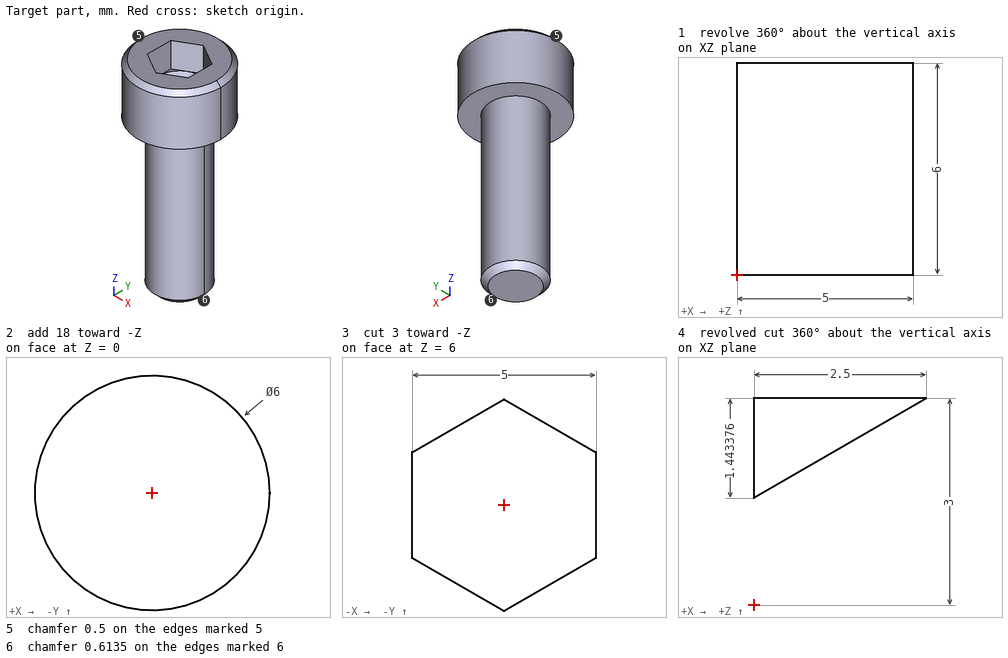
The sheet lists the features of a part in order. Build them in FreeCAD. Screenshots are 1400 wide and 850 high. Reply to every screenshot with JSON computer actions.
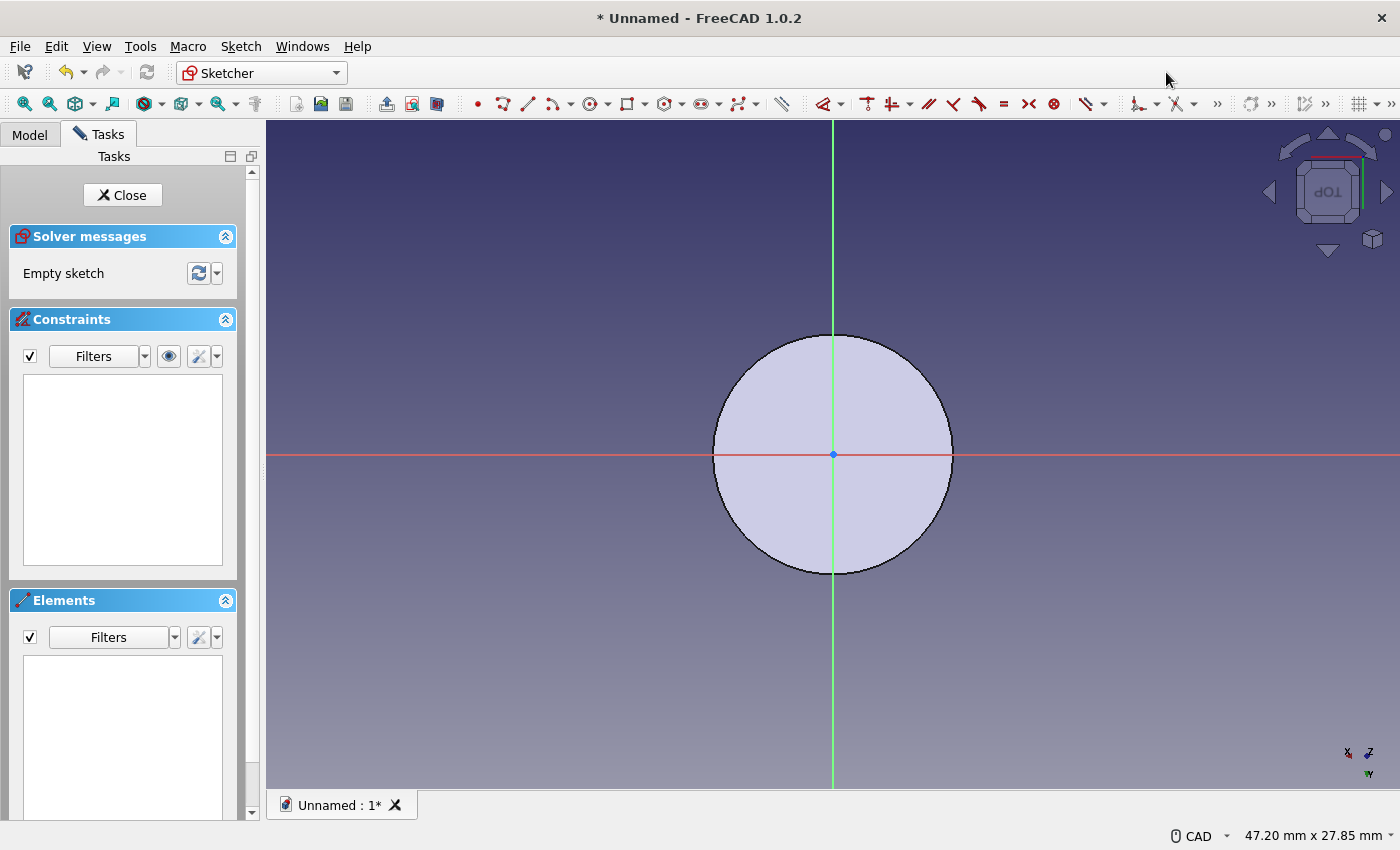
{"action": "scroll", "coordinate": [863, 454], "scroll_direction": "up", "scroll_amount": 6}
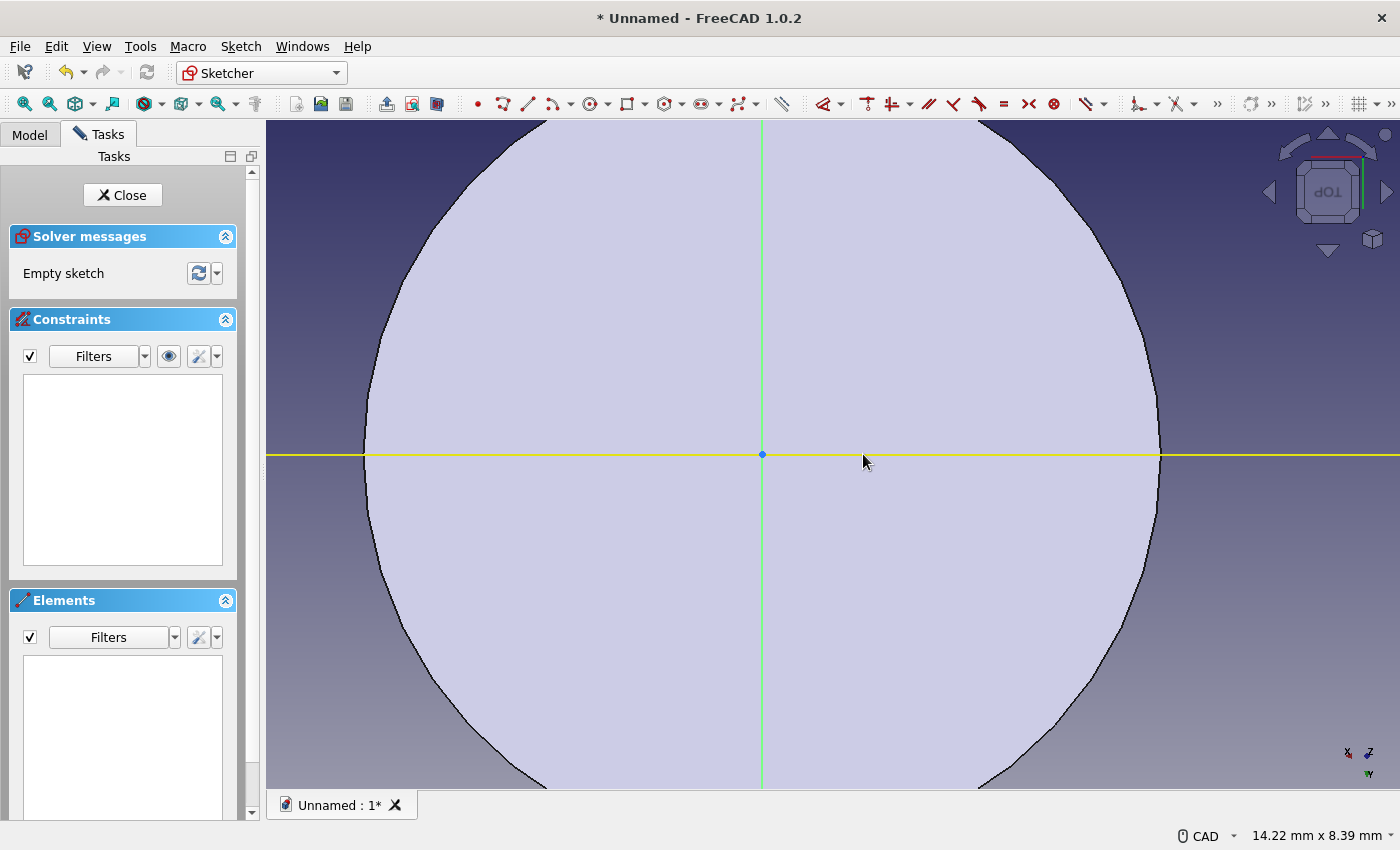
{"action": "left_click", "coordinate": [664, 104]}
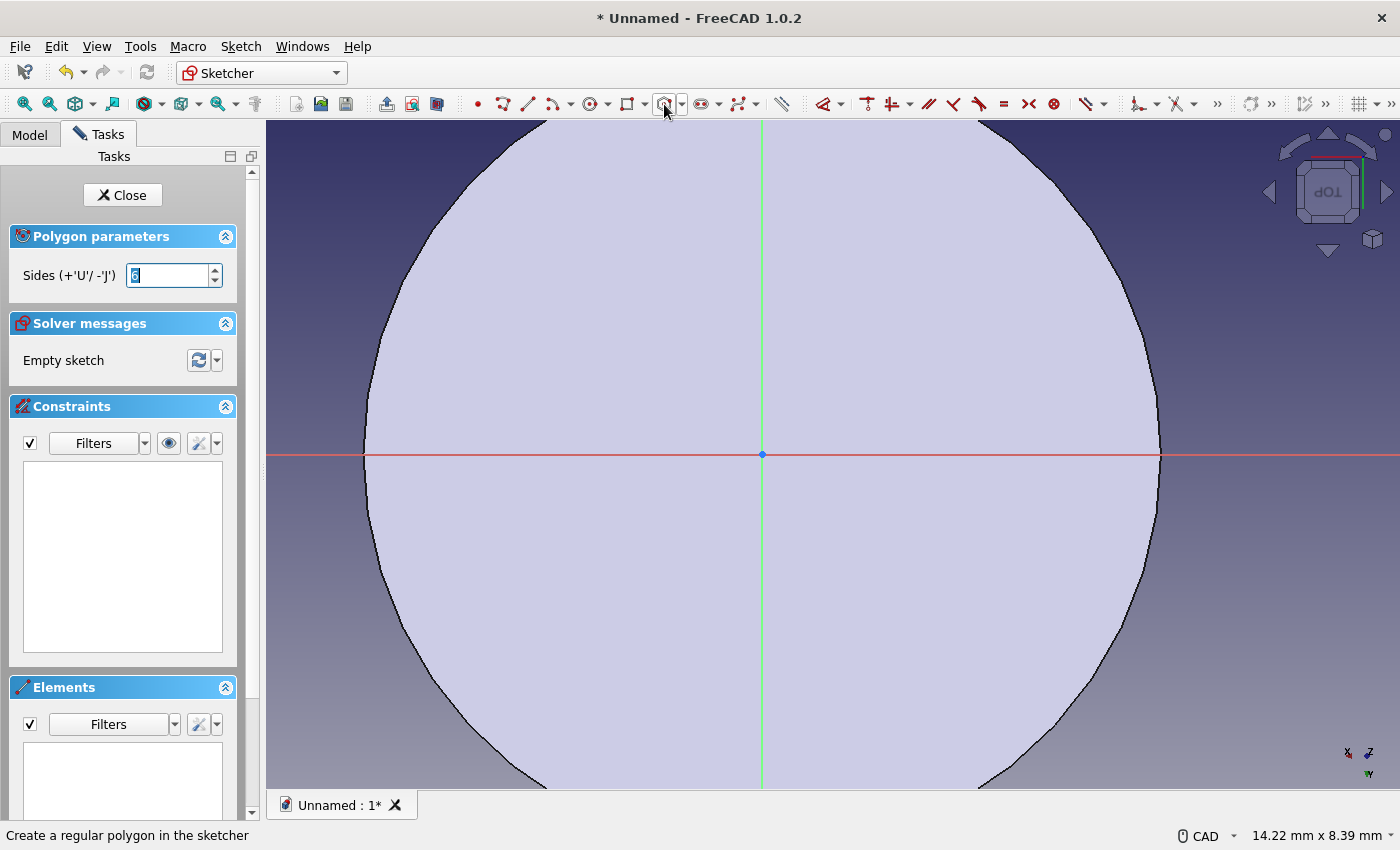
{"action": "left_click", "coordinate": [762, 454]}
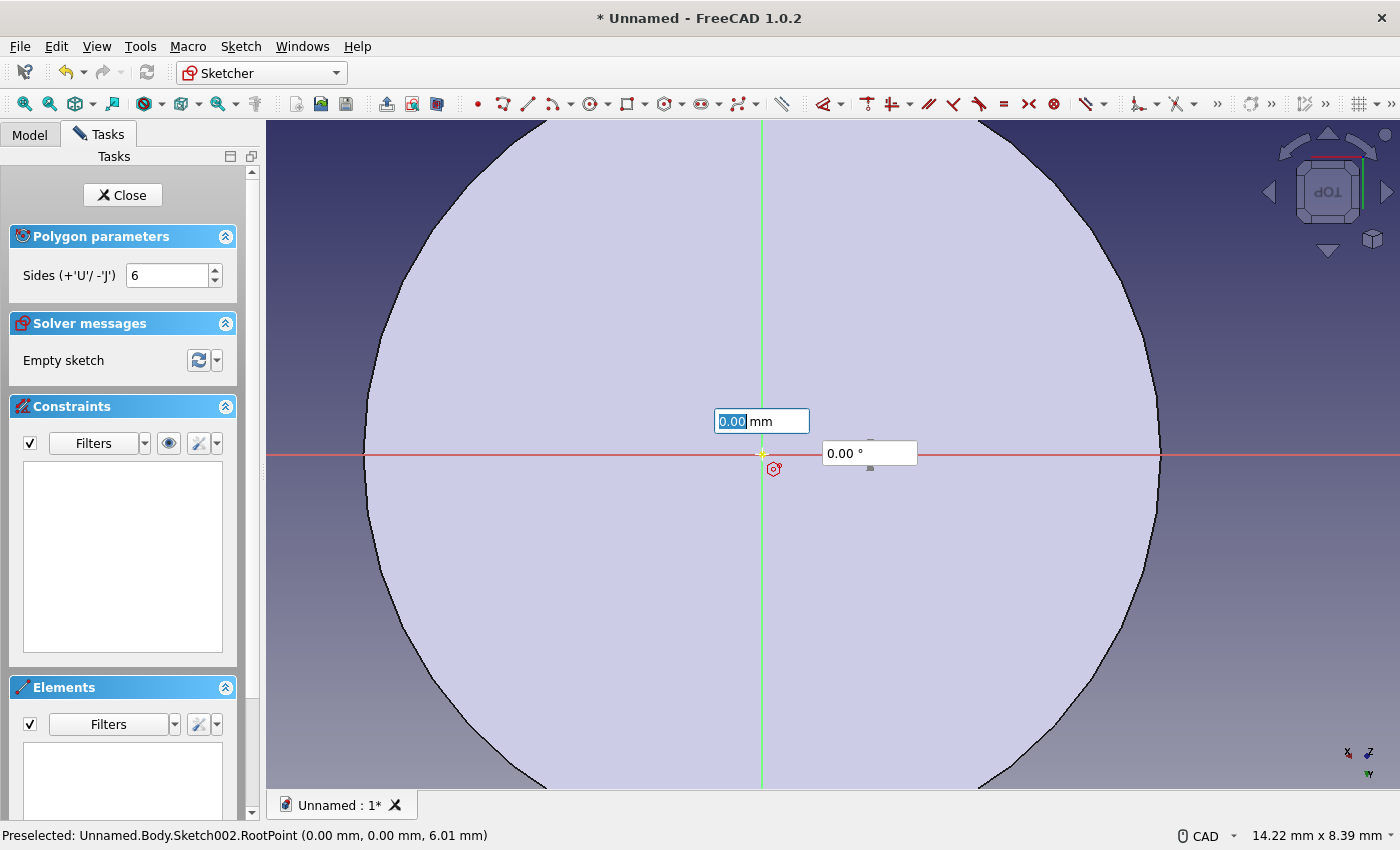
{"action": "left_click", "coordinate": [762, 685]}
{"action": "right_click", "coordinate": [762, 685]}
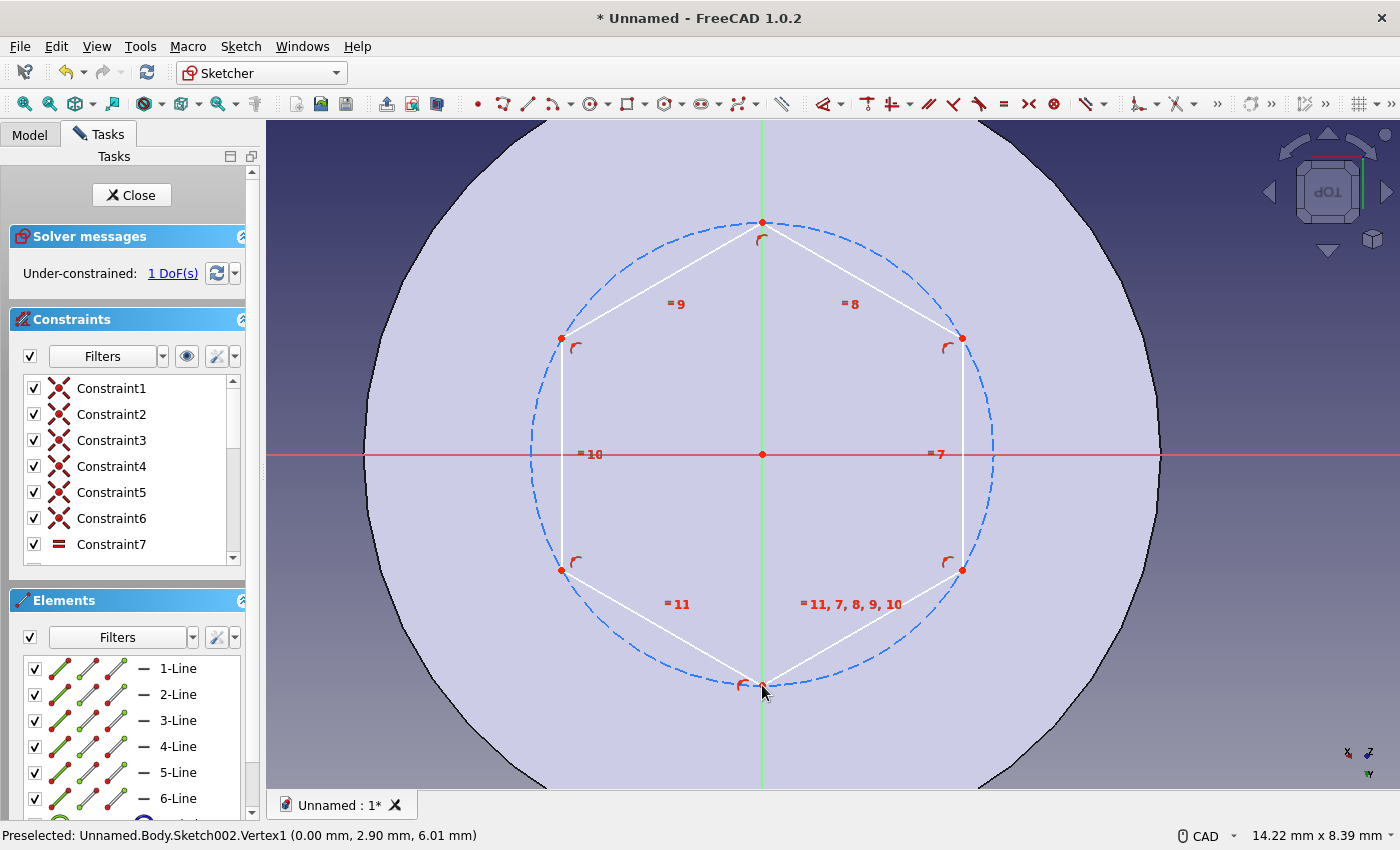
{"action": "left_click", "coordinate": [822, 104]}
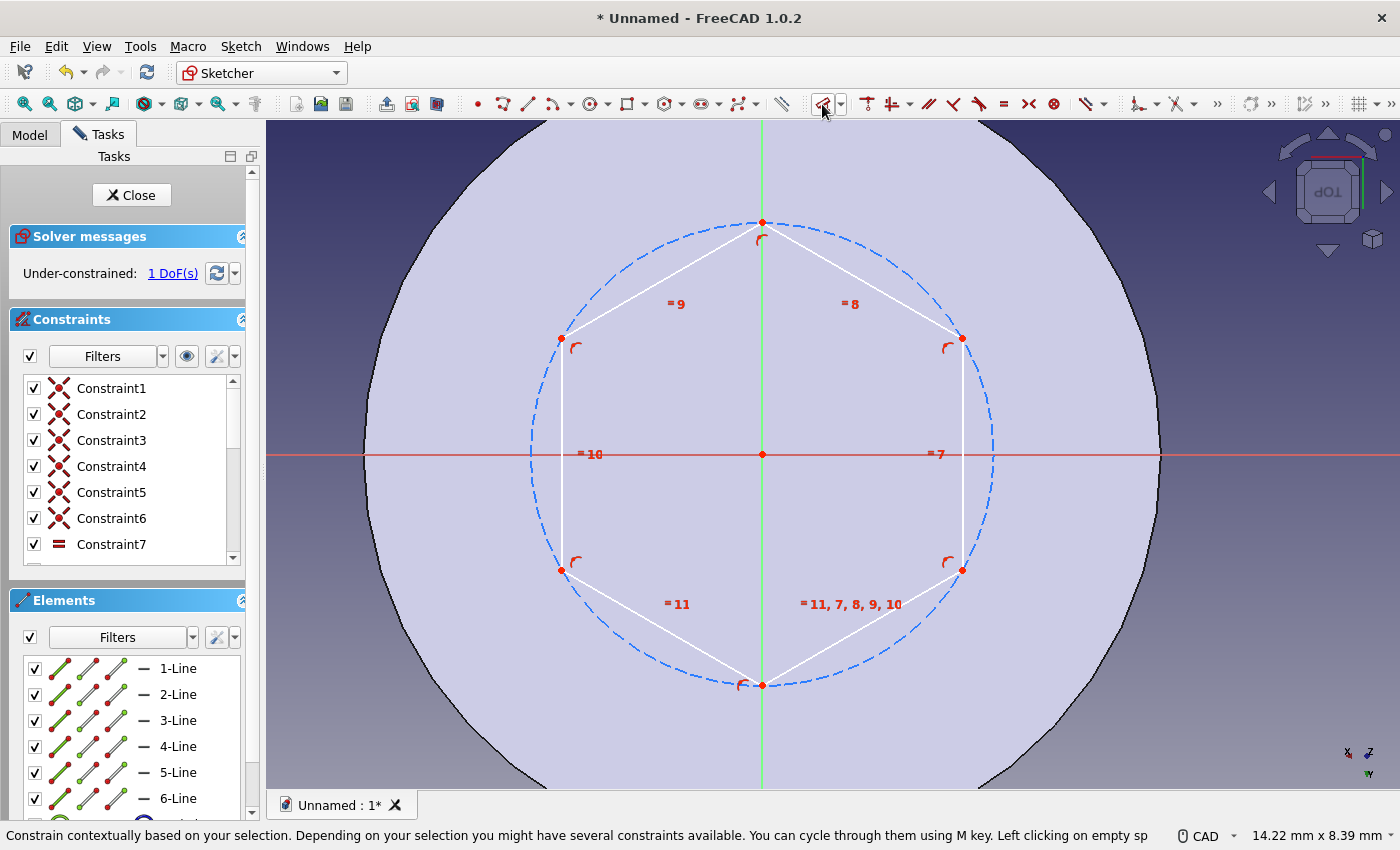
{"action": "left_click", "coordinate": [562, 339]}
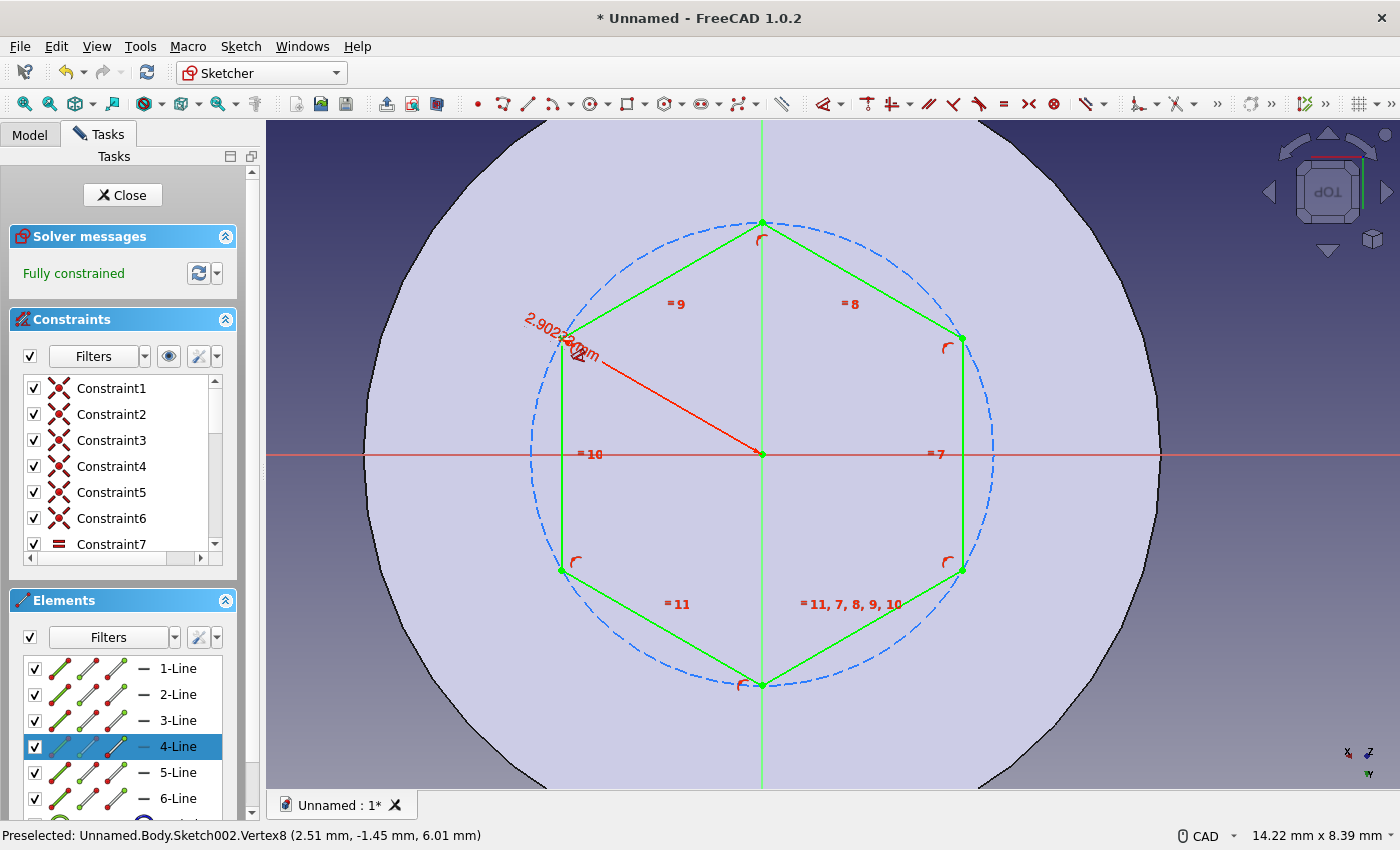
{"action": "left_click", "coordinate": [963, 570]}
{"action": "left_click", "coordinate": [670, 305]}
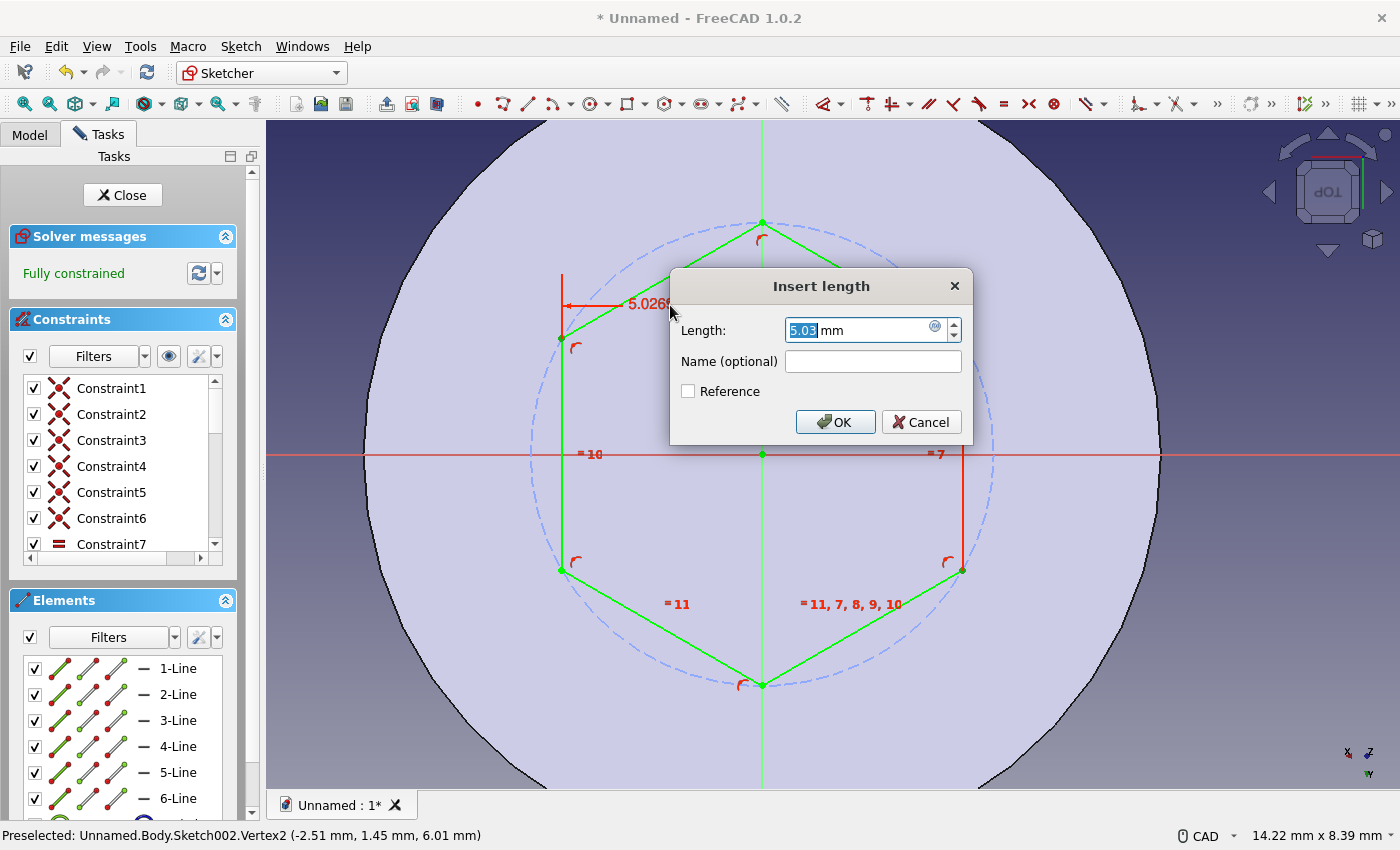
{"action": "type", "text": "5"}
{"action": "key", "text": "Return"}
{"action": "key", "text": "Escape"}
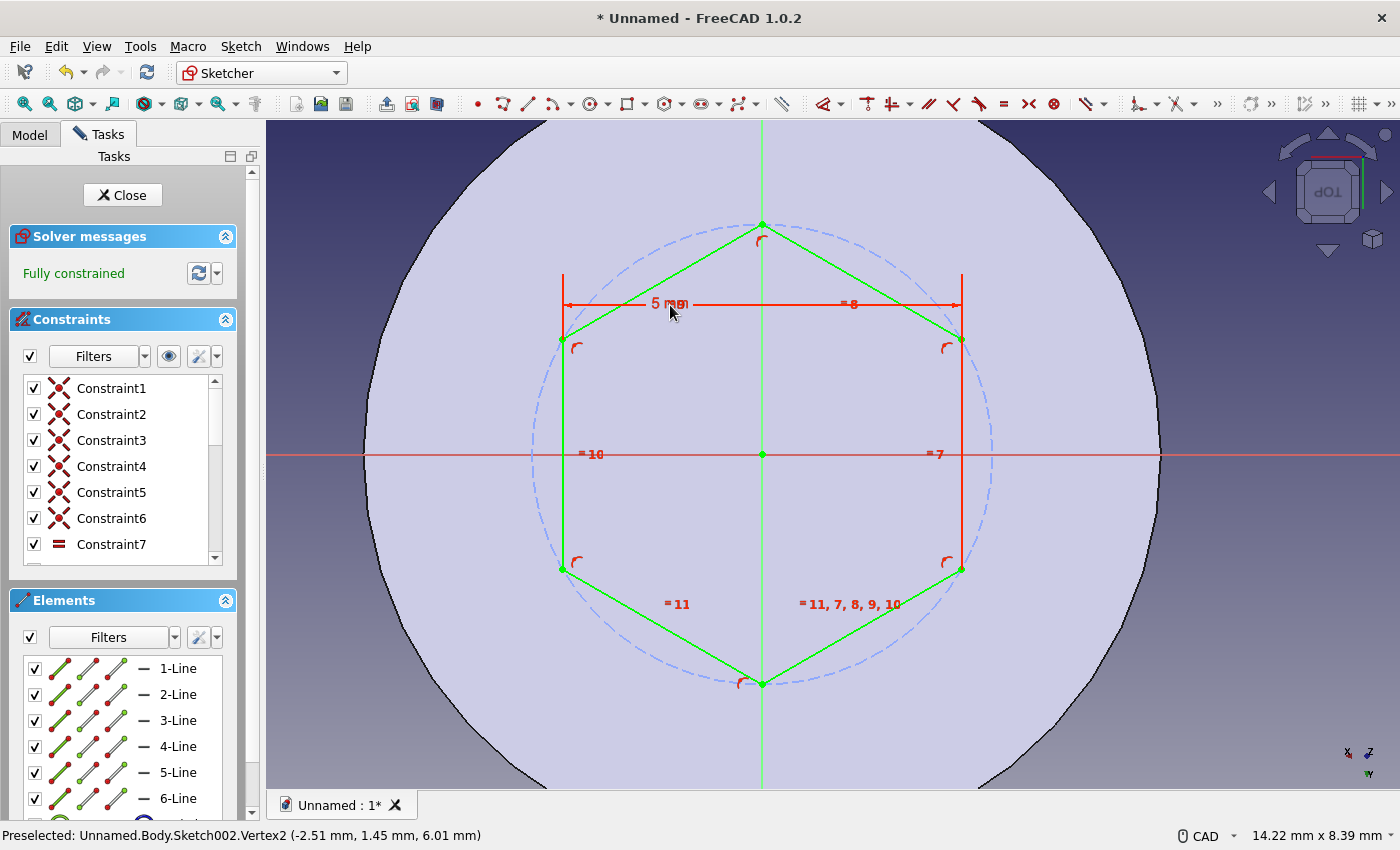
{"action": "left_click", "coordinate": [123, 195]}